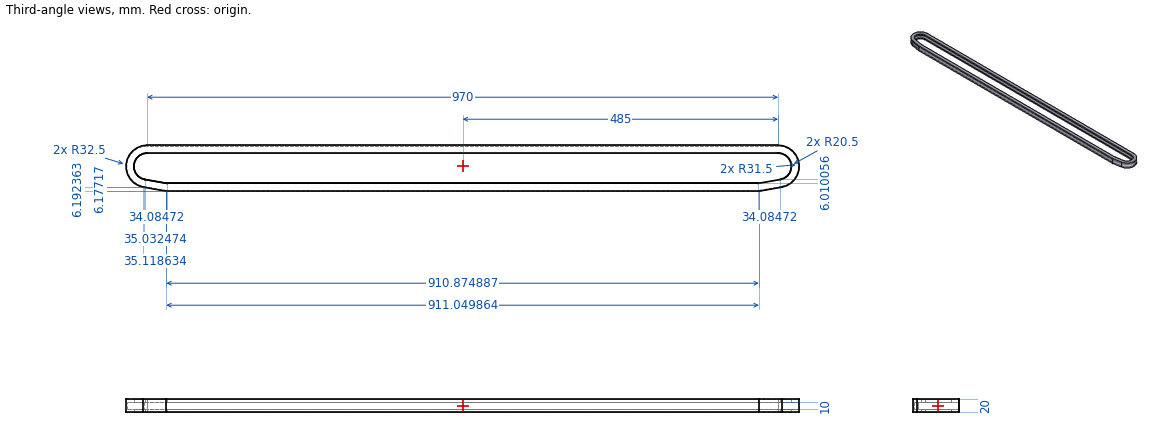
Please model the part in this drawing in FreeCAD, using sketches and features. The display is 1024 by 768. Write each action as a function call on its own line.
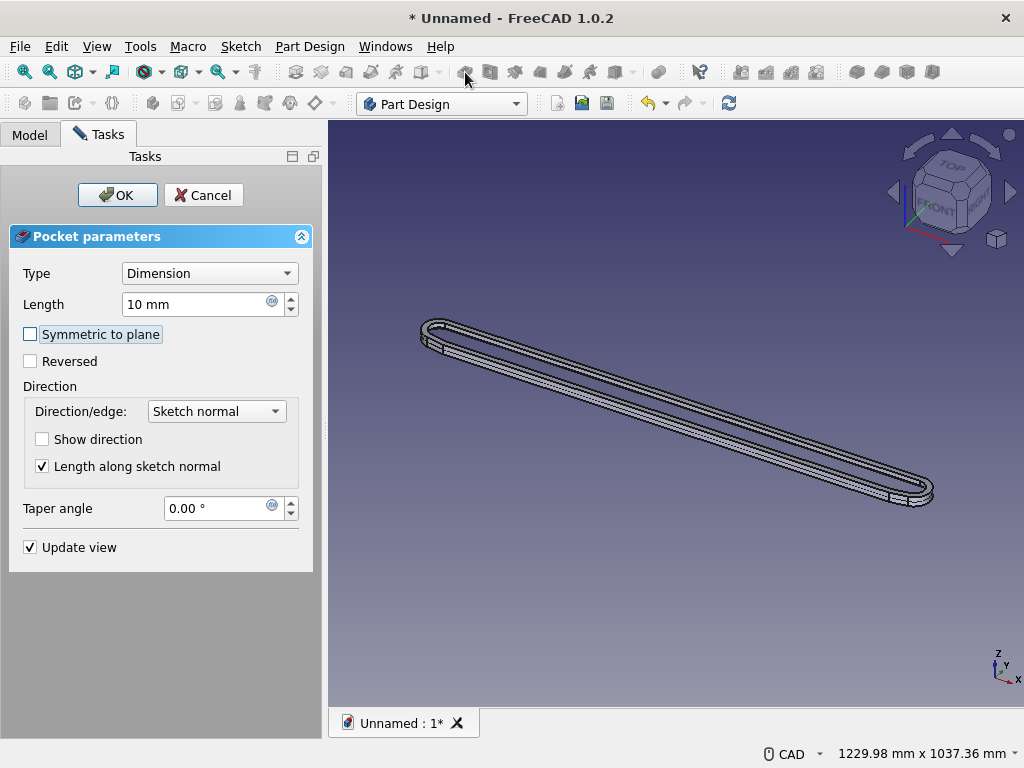
click(31, 334)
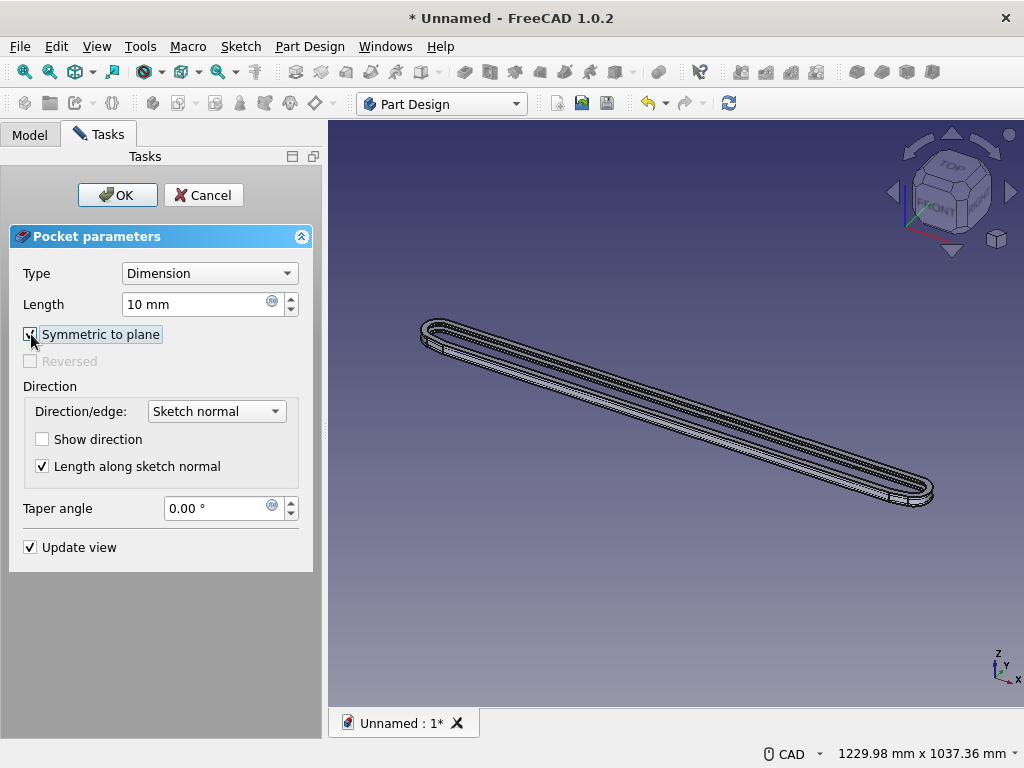
click(118, 195)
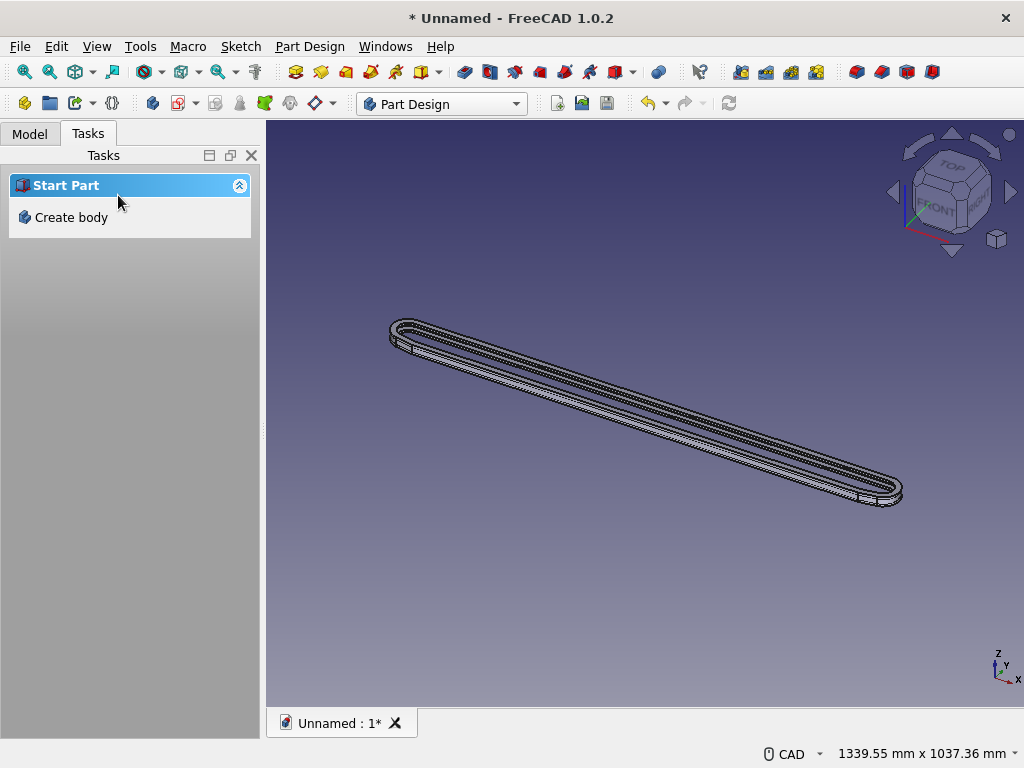
key(0)